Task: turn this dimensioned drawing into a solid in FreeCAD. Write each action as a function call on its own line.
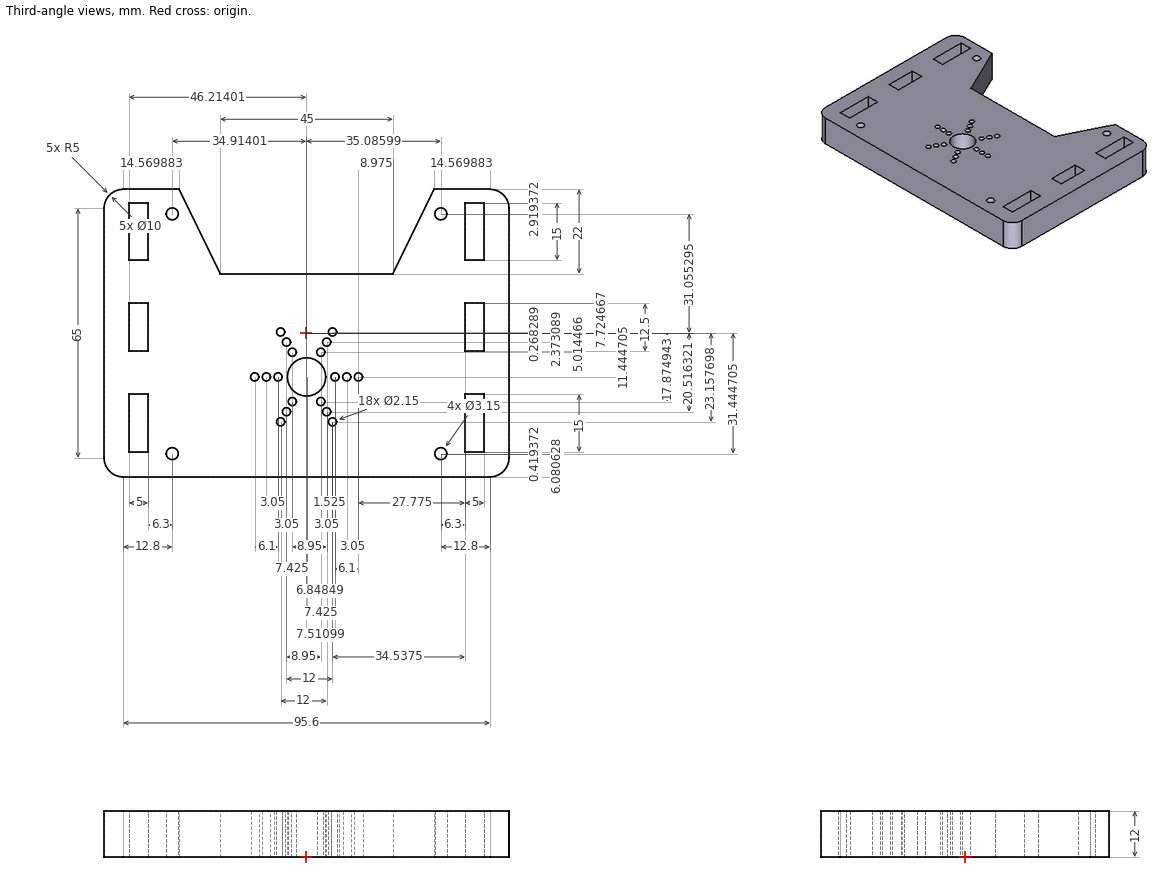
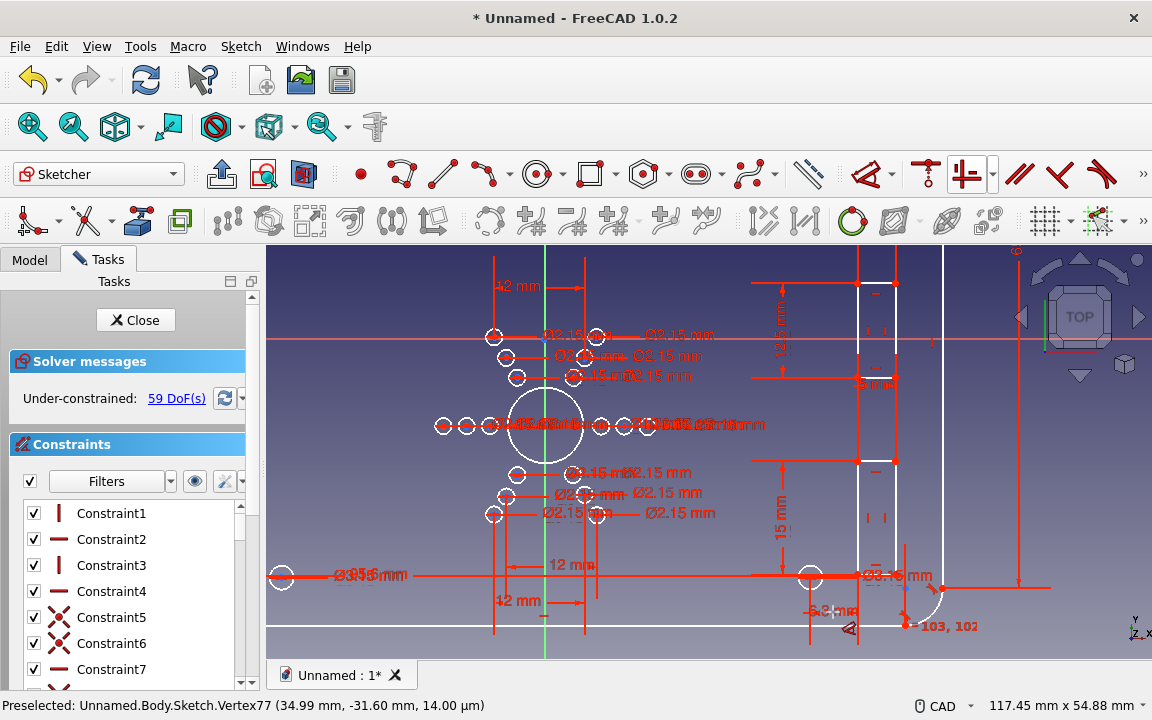
click(647, 427)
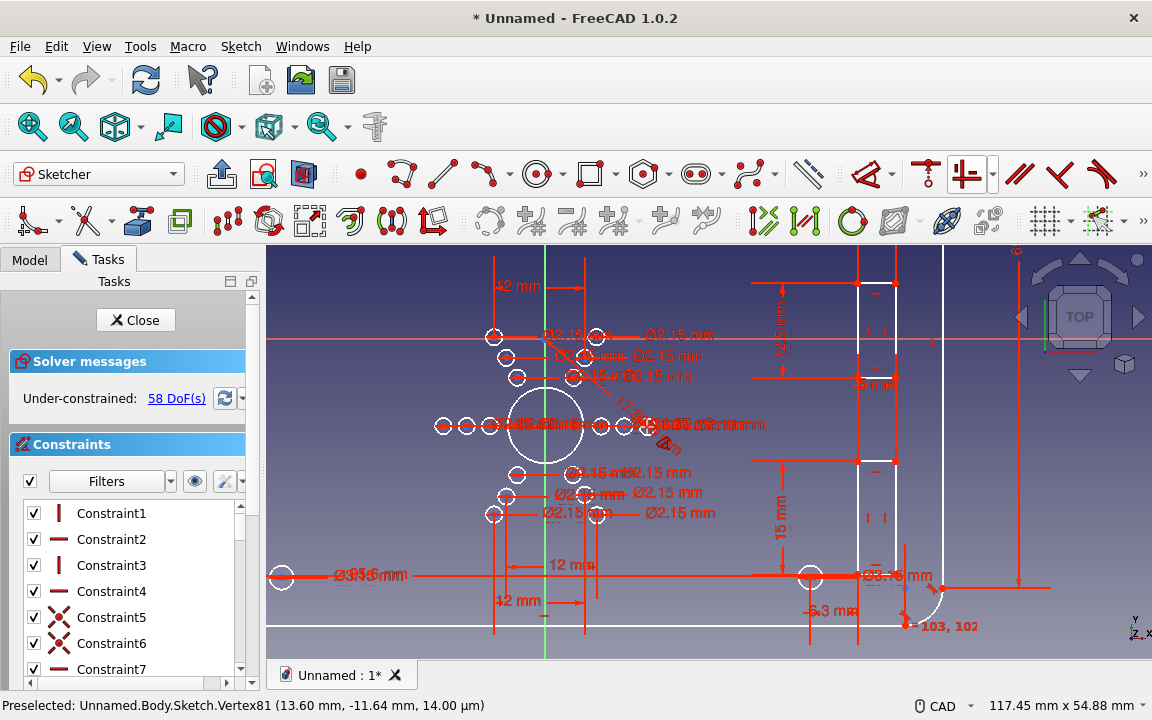
click(601, 426)
click(624, 461)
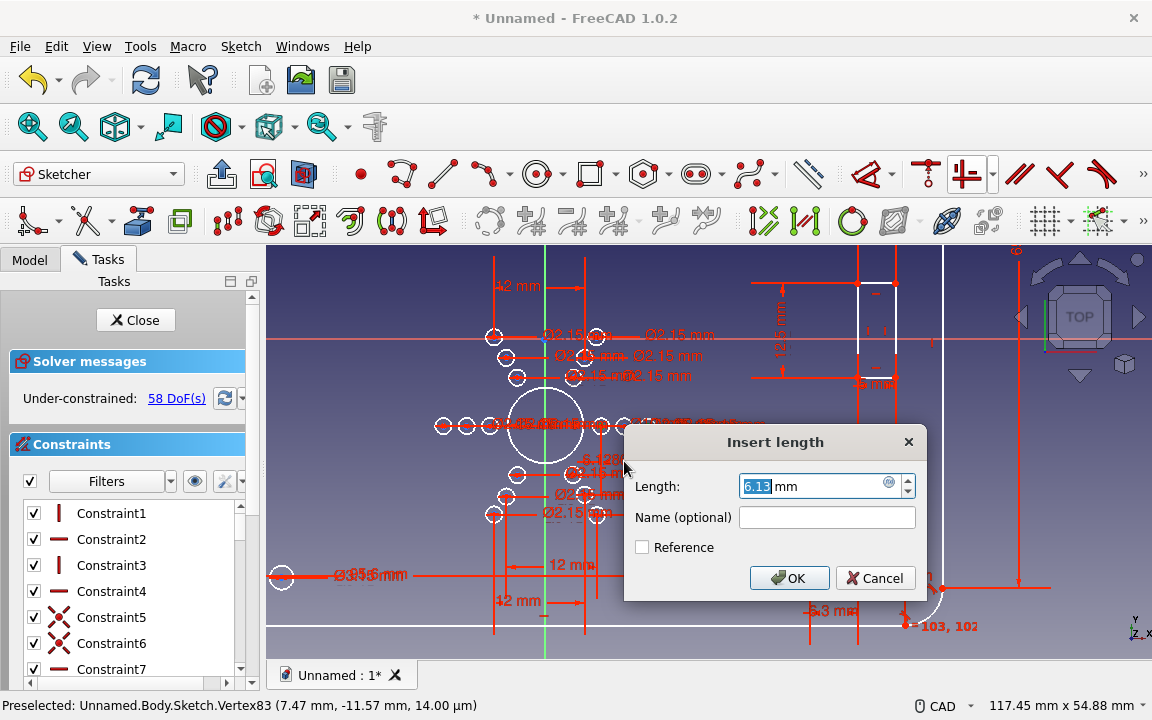
text(6.1)
key(Return)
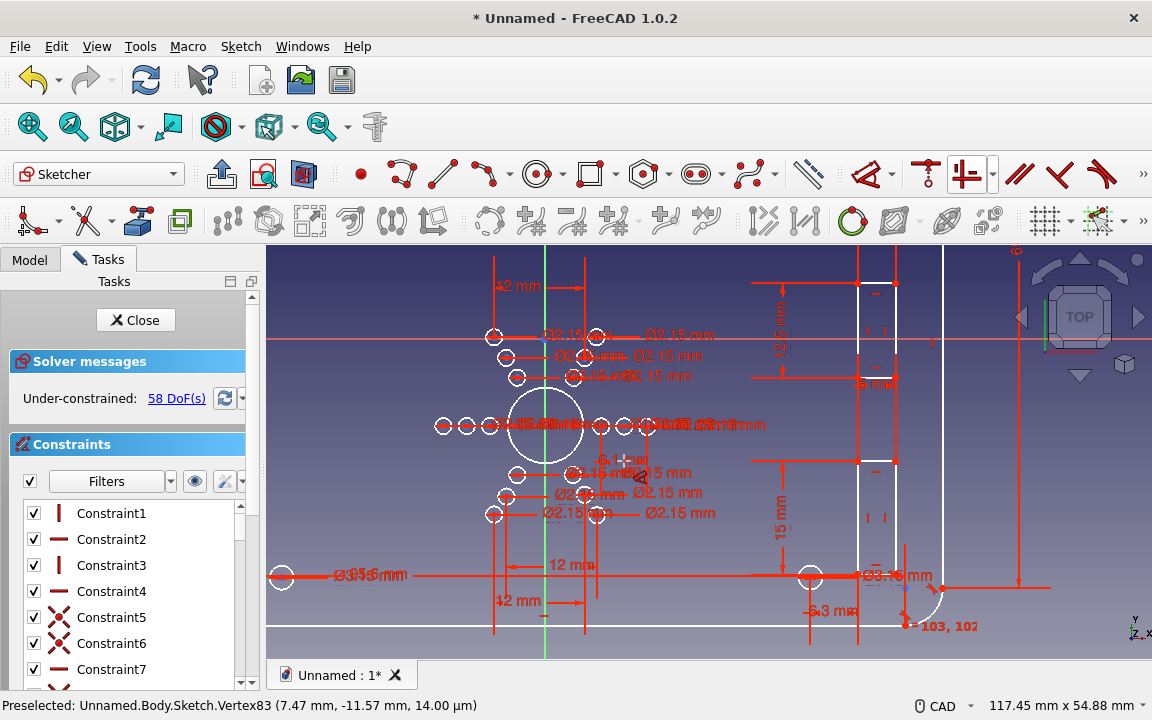
scroll(718, 544, down, 4)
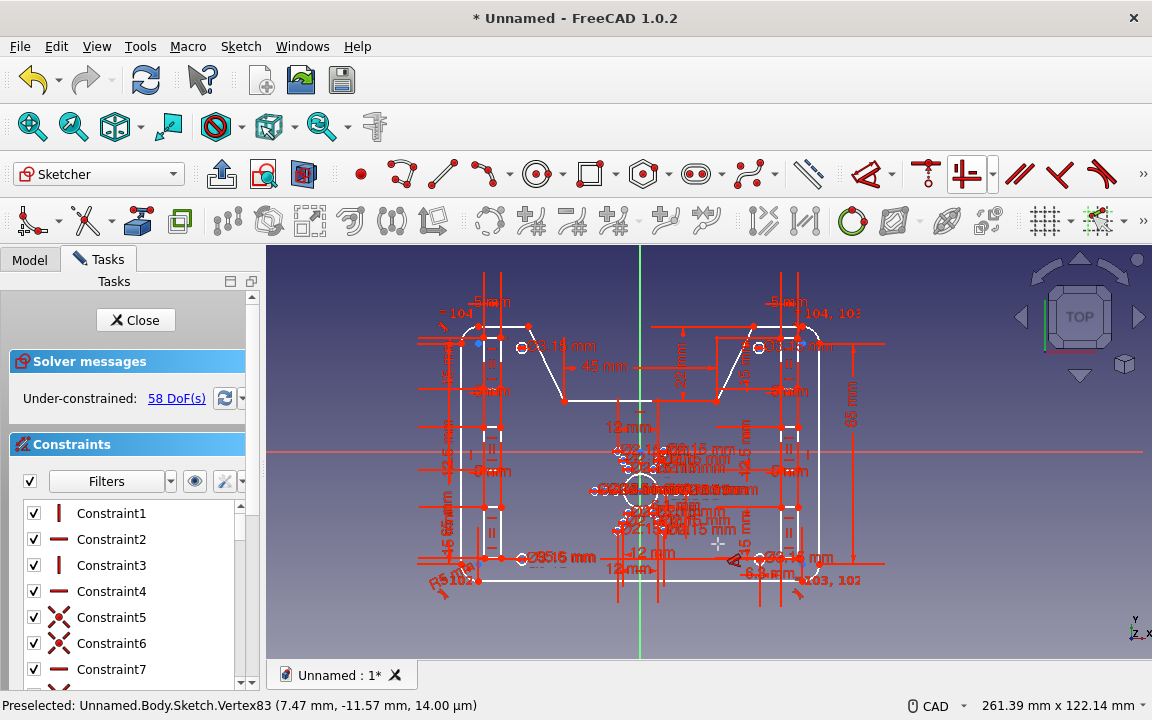
scroll(501, 558, up, 4)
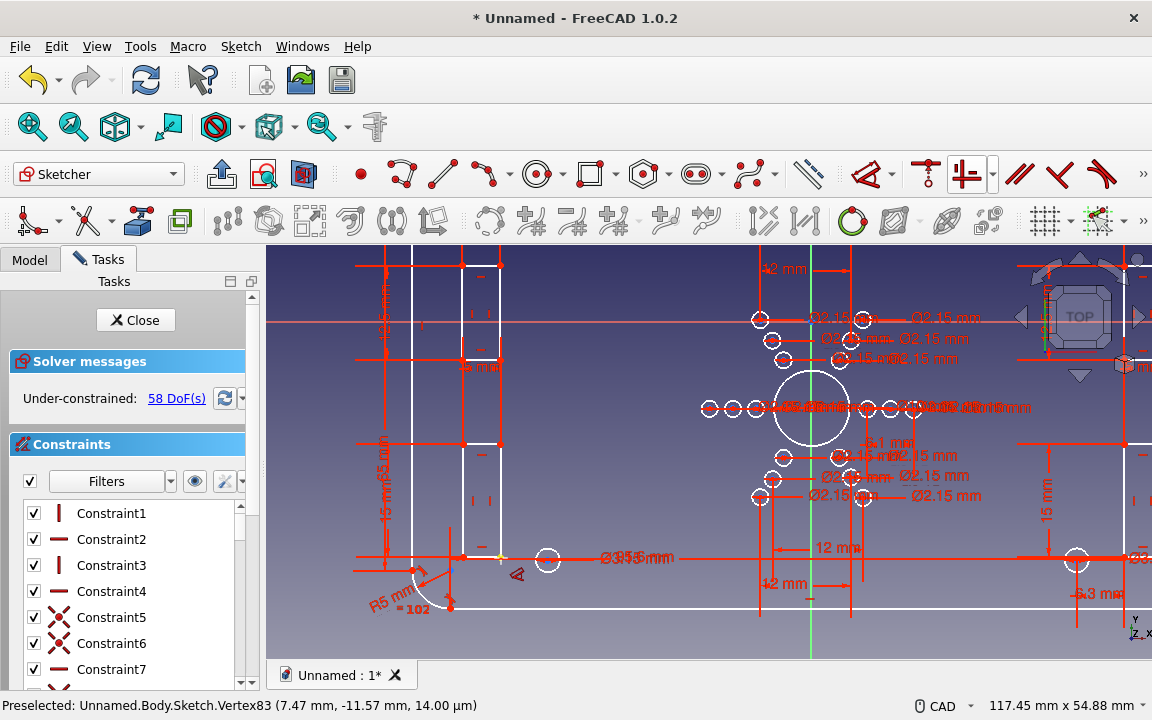
click(501, 557)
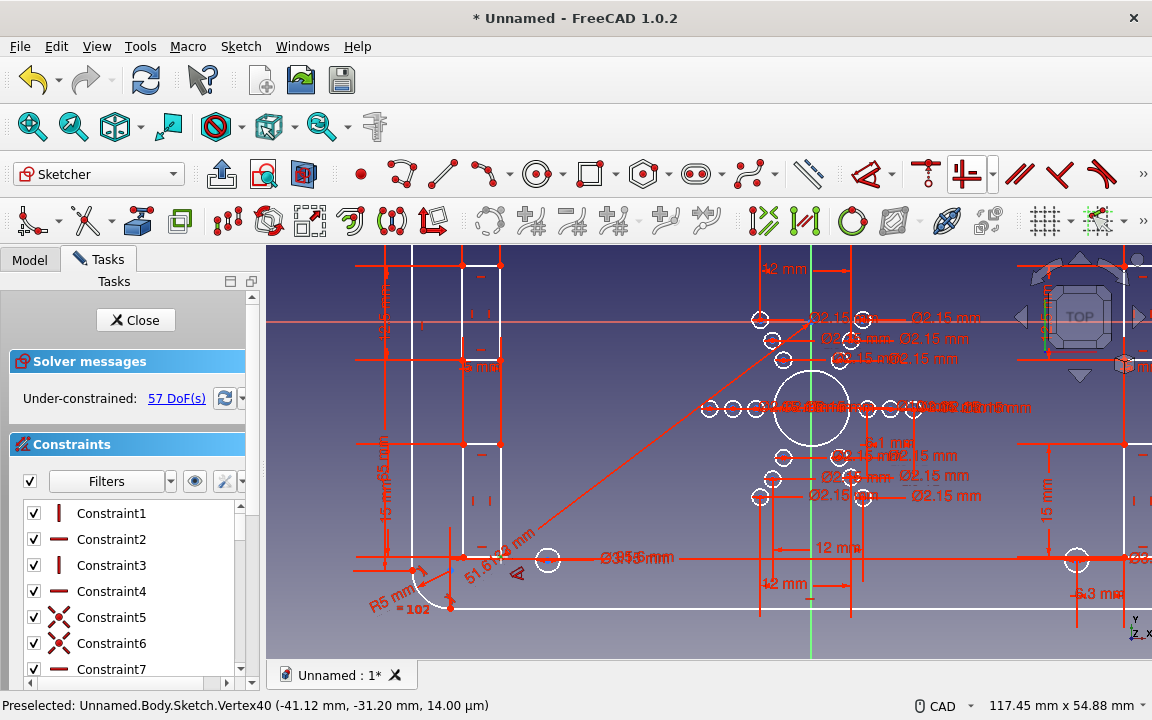
click(548, 560)
click(524, 594)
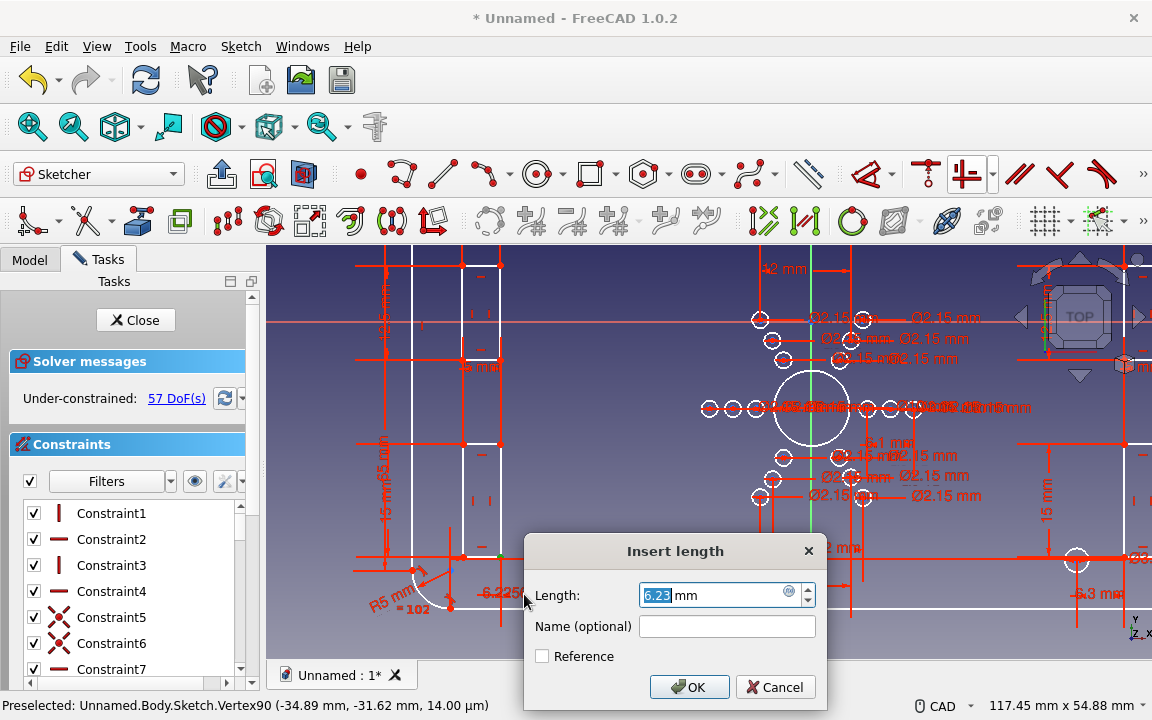
text(6.3)
key(Return)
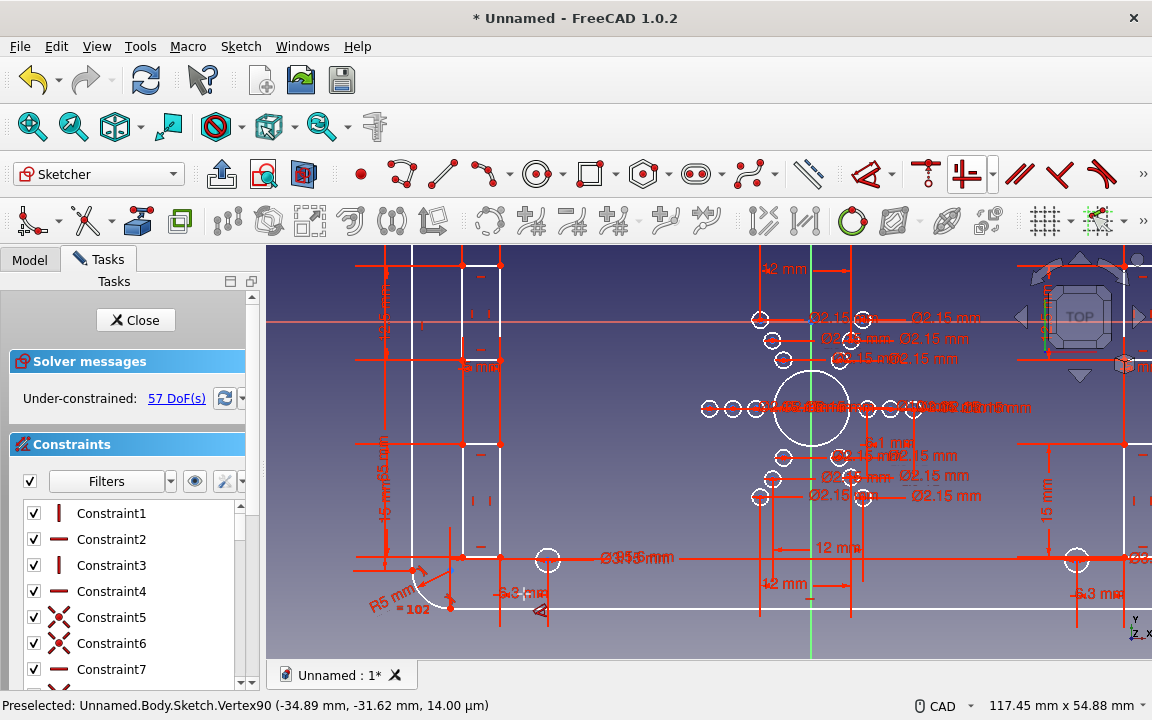
click(756, 409)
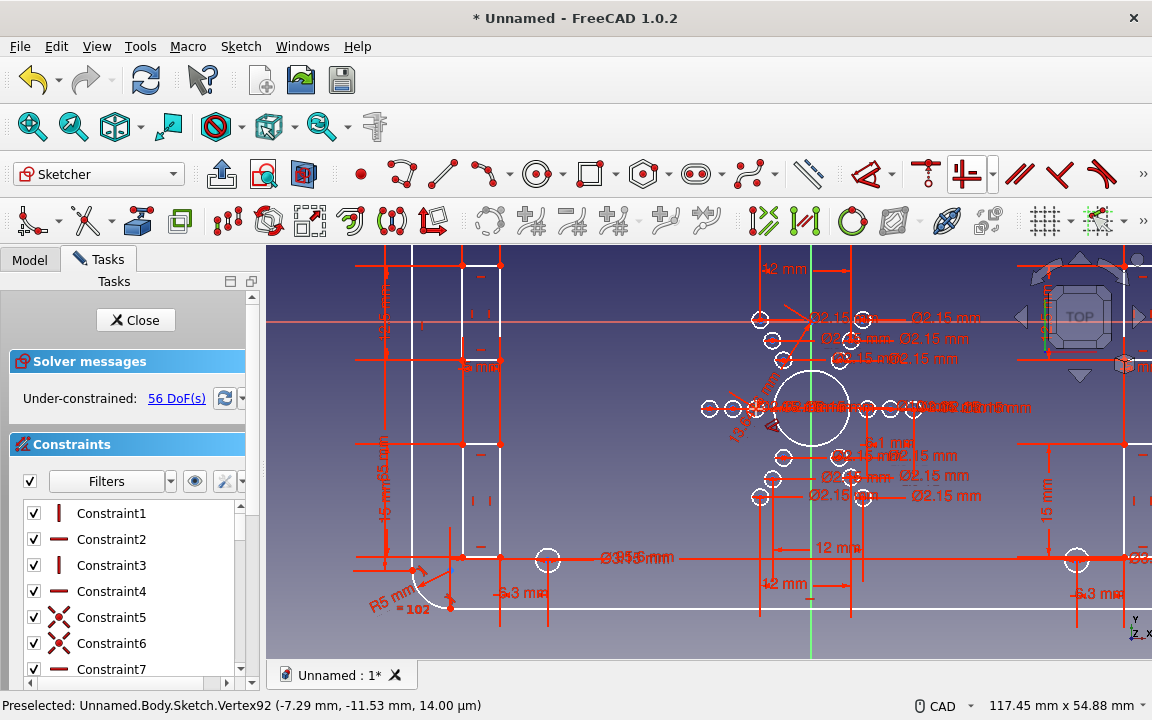
click(710, 409)
click(733, 443)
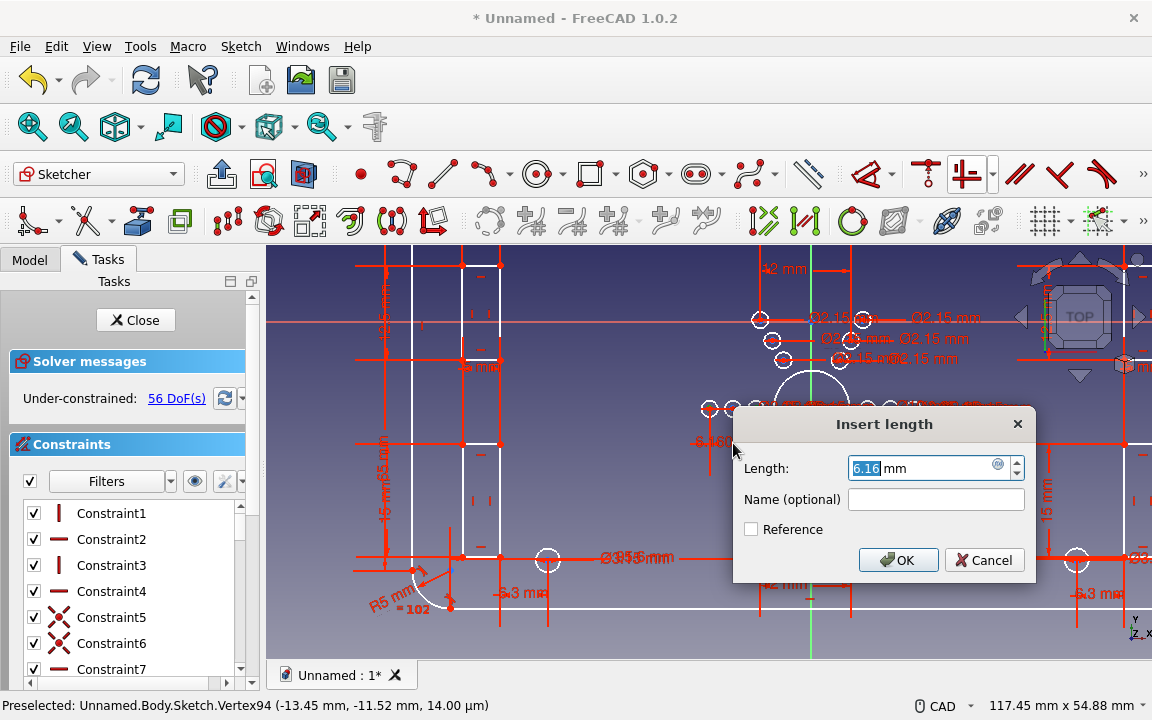
text(6.1)
key(Return)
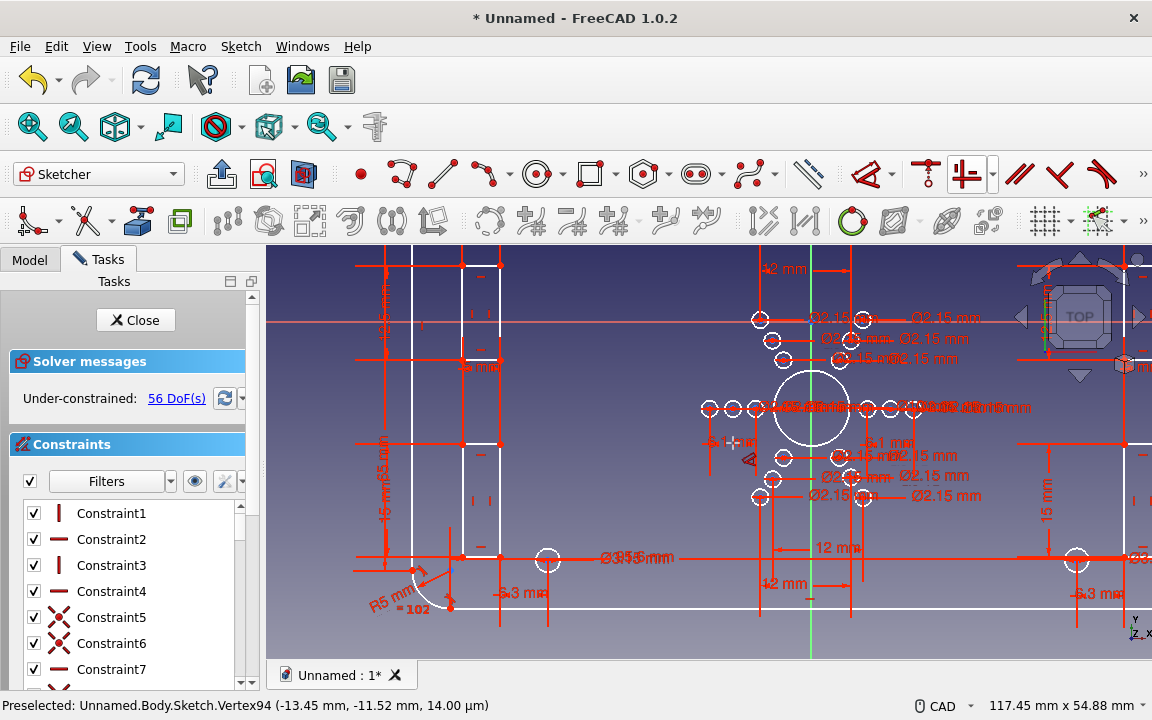
scroll(501, 558, down, 4)